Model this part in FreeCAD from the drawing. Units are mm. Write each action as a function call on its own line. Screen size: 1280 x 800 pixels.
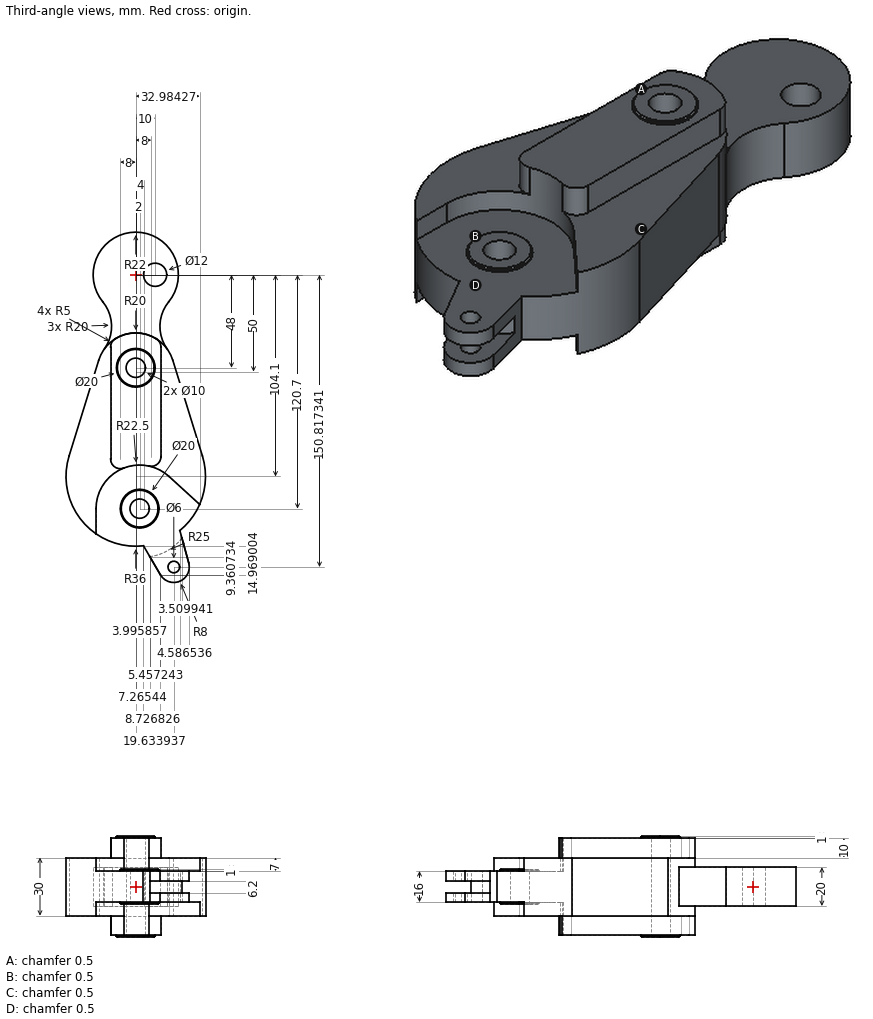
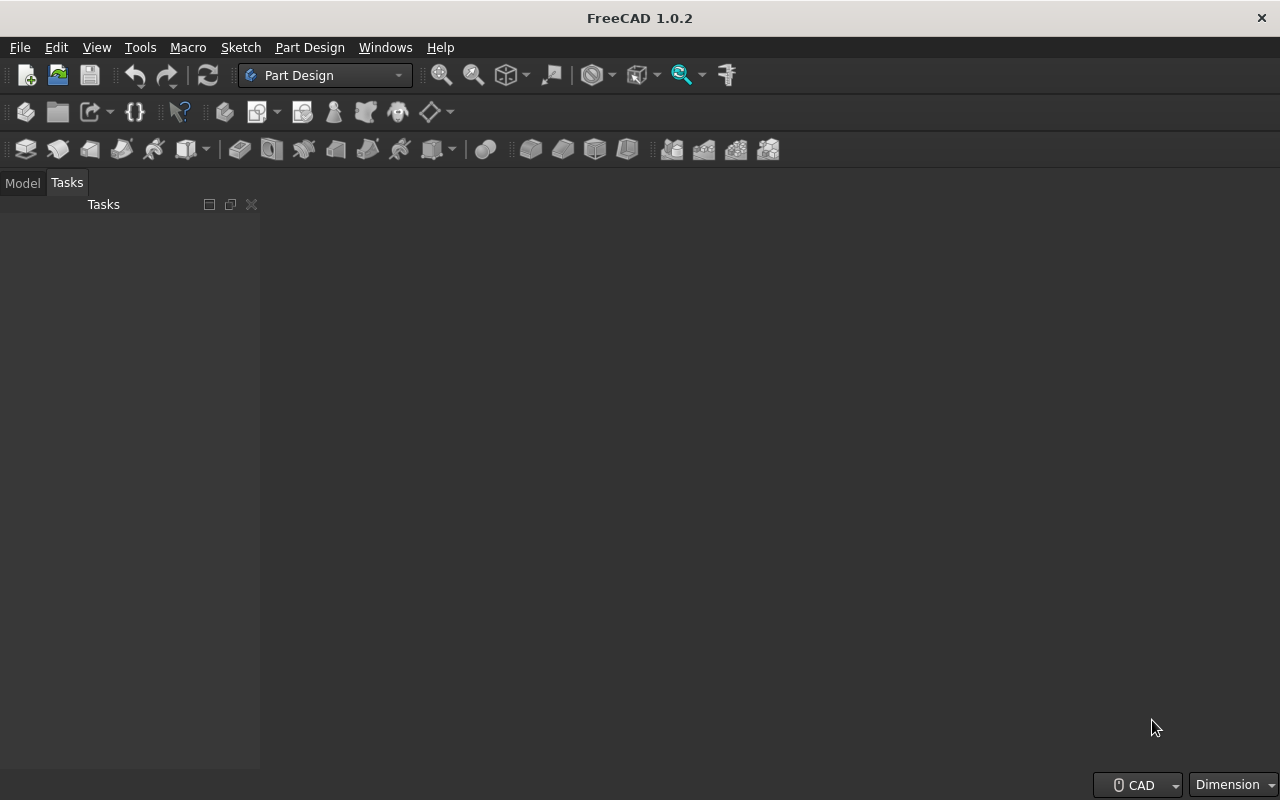
click(26, 76)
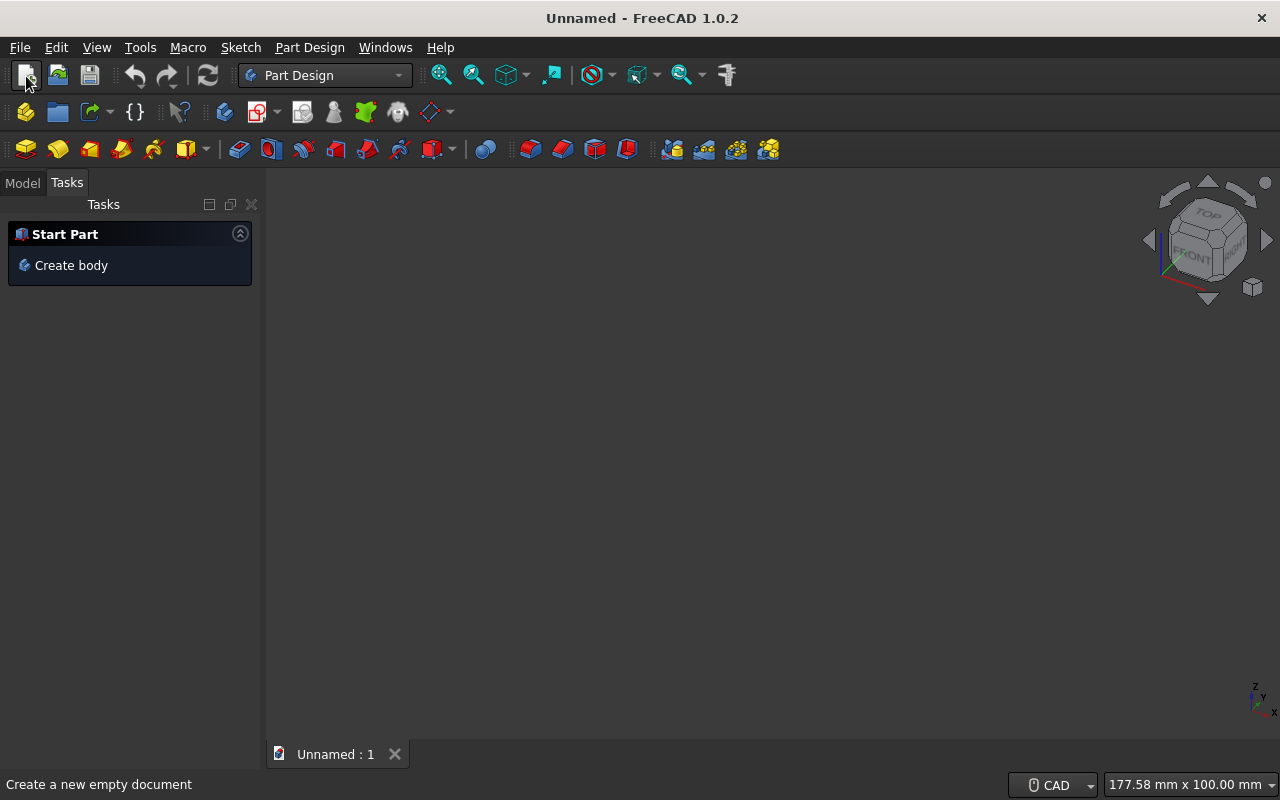
click(258, 112)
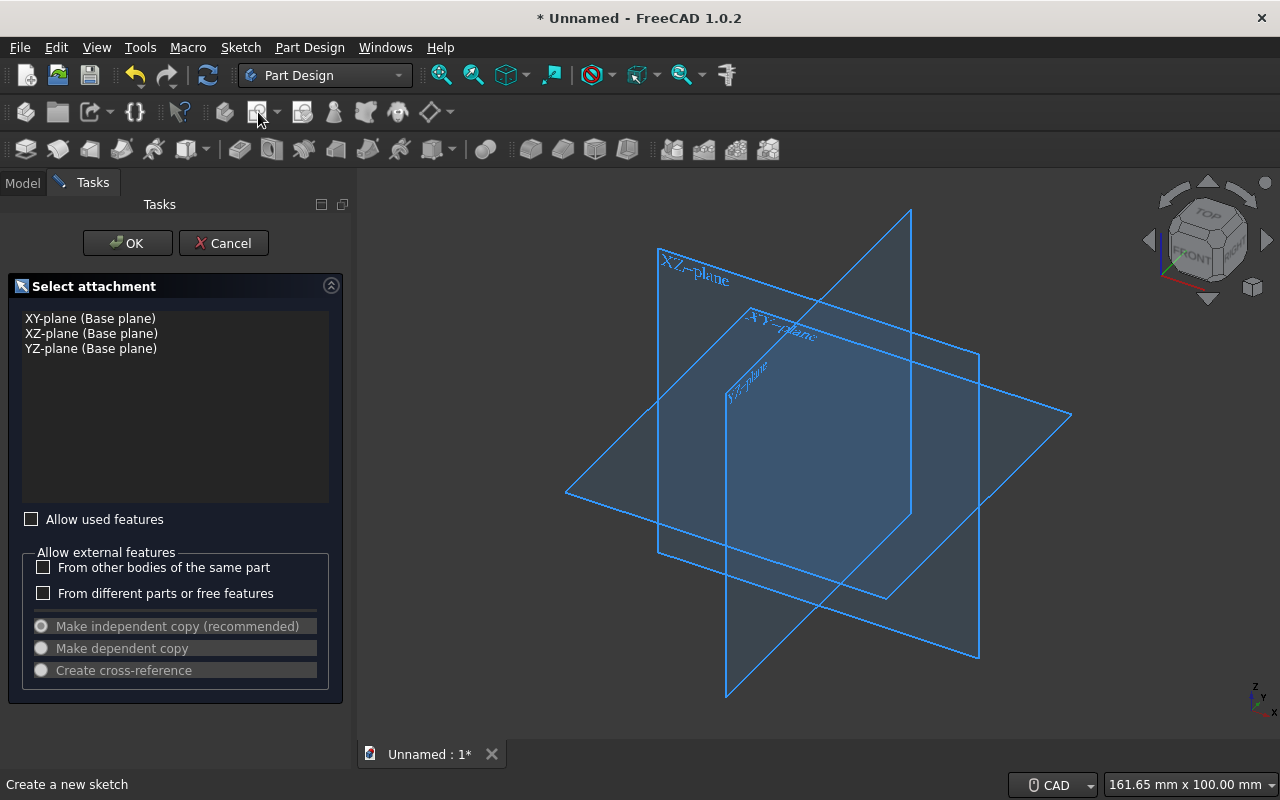
click(82, 318)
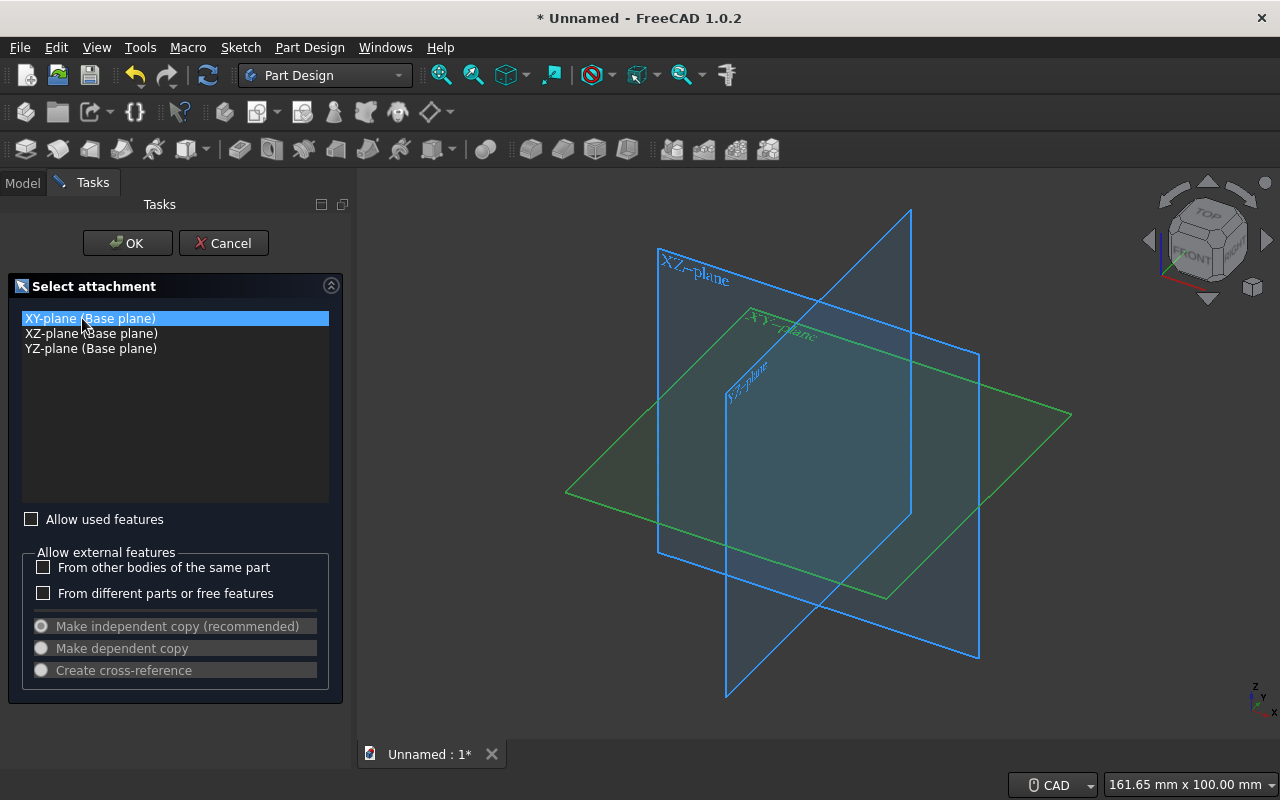
click(128, 243)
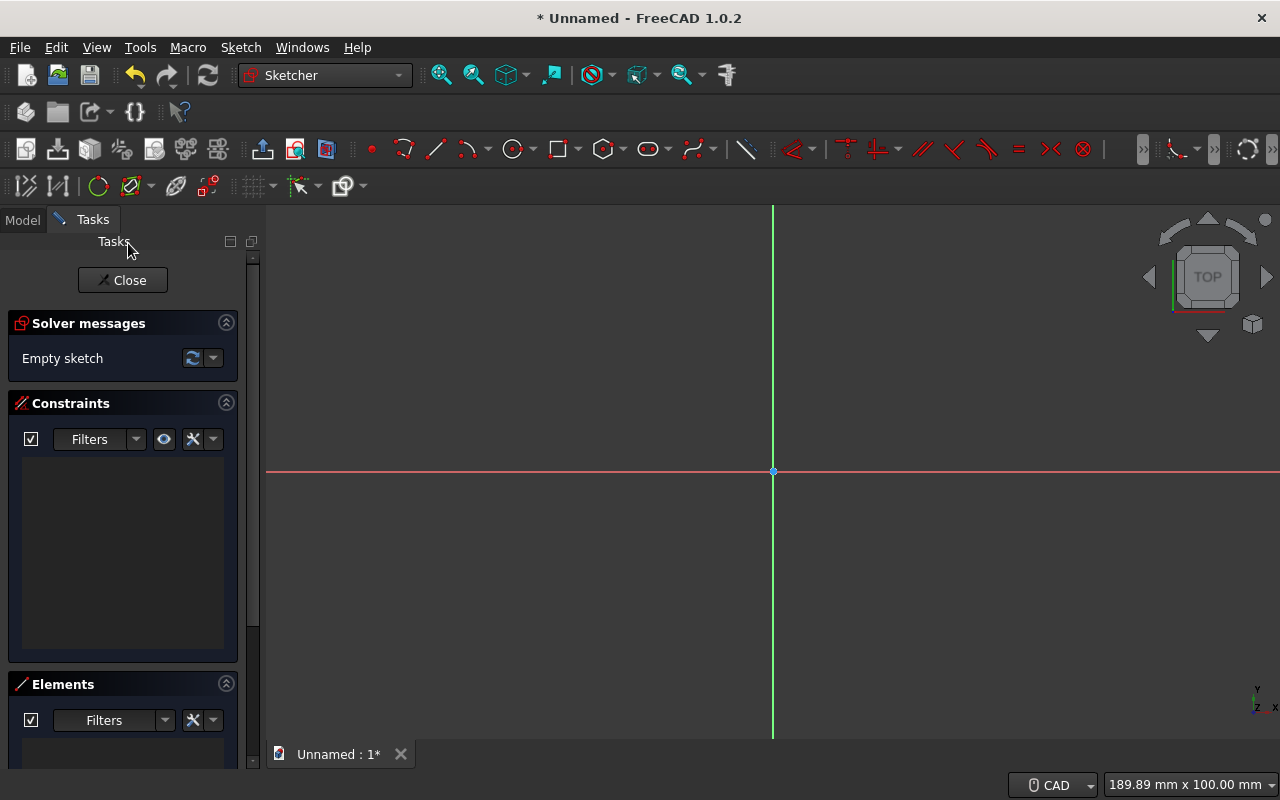
click(490, 150)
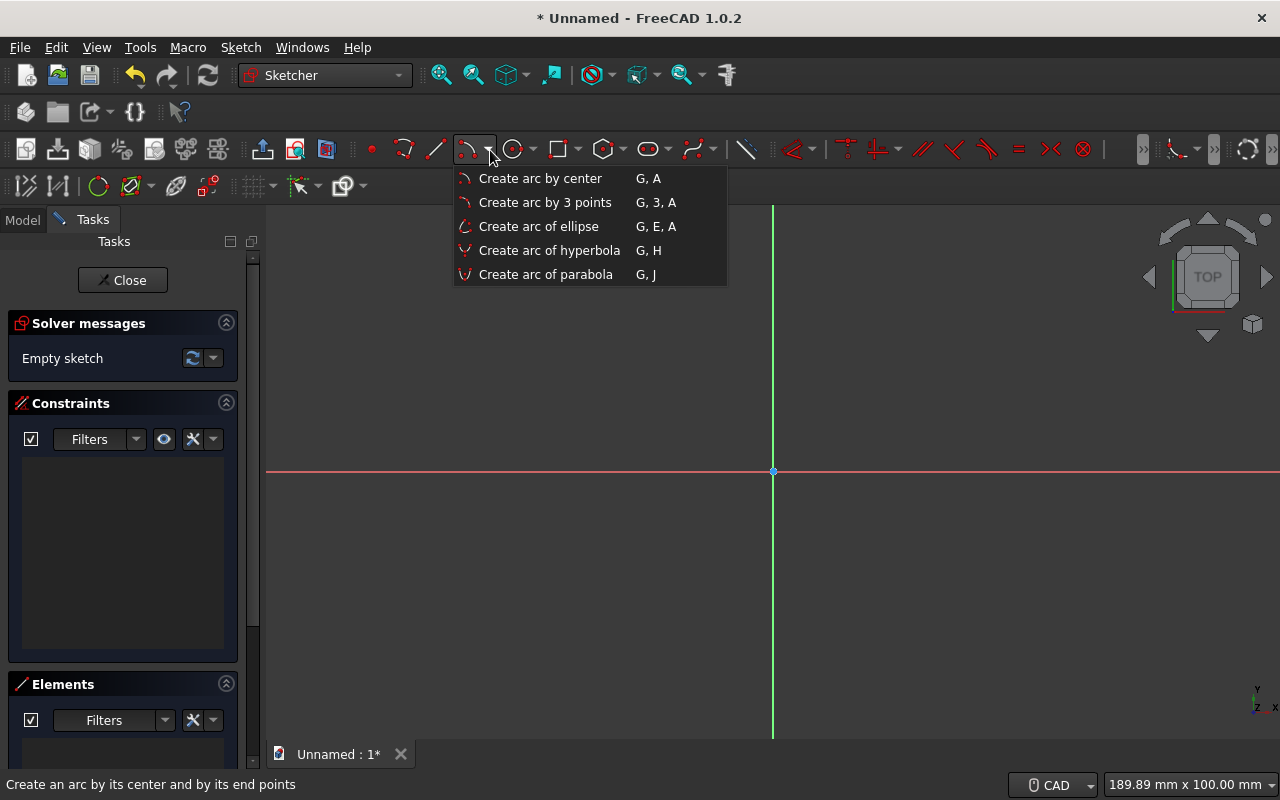
click(590, 202)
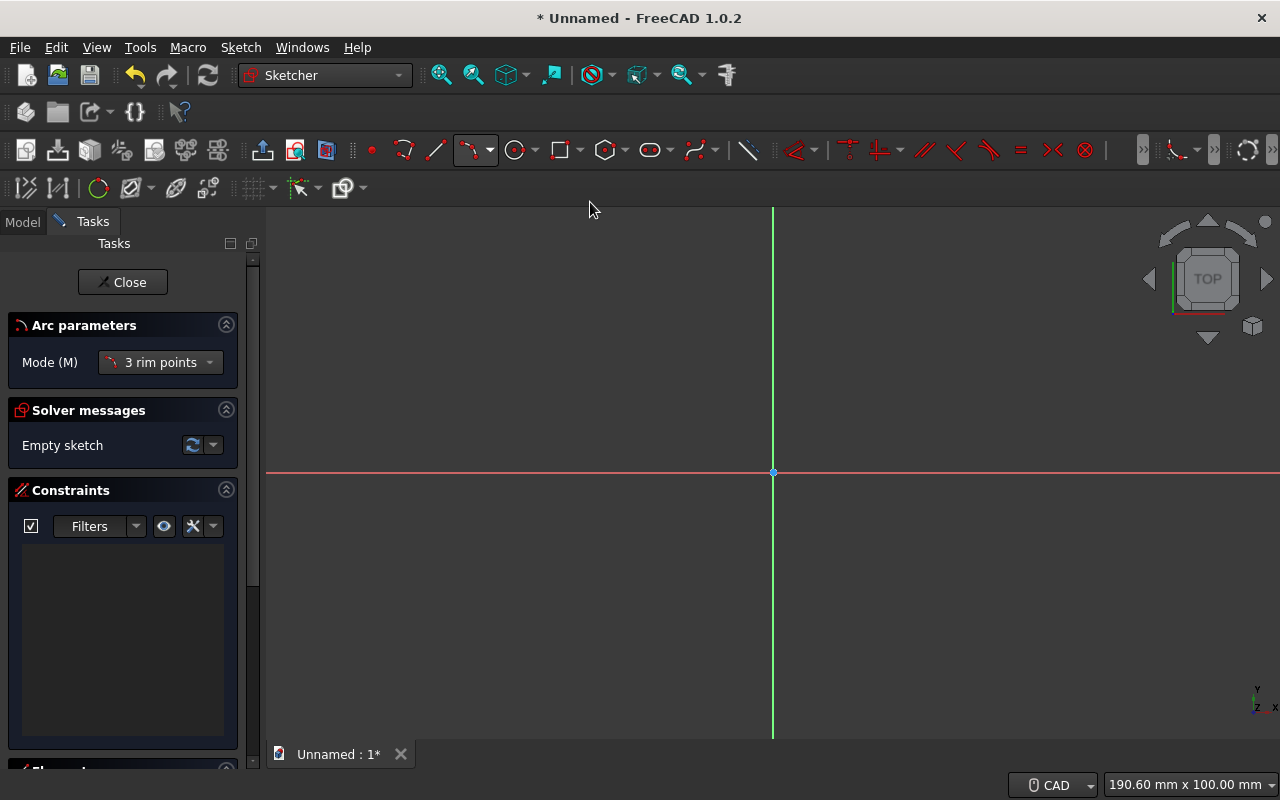
click(683, 547)
click(687, 677)
click(707, 611)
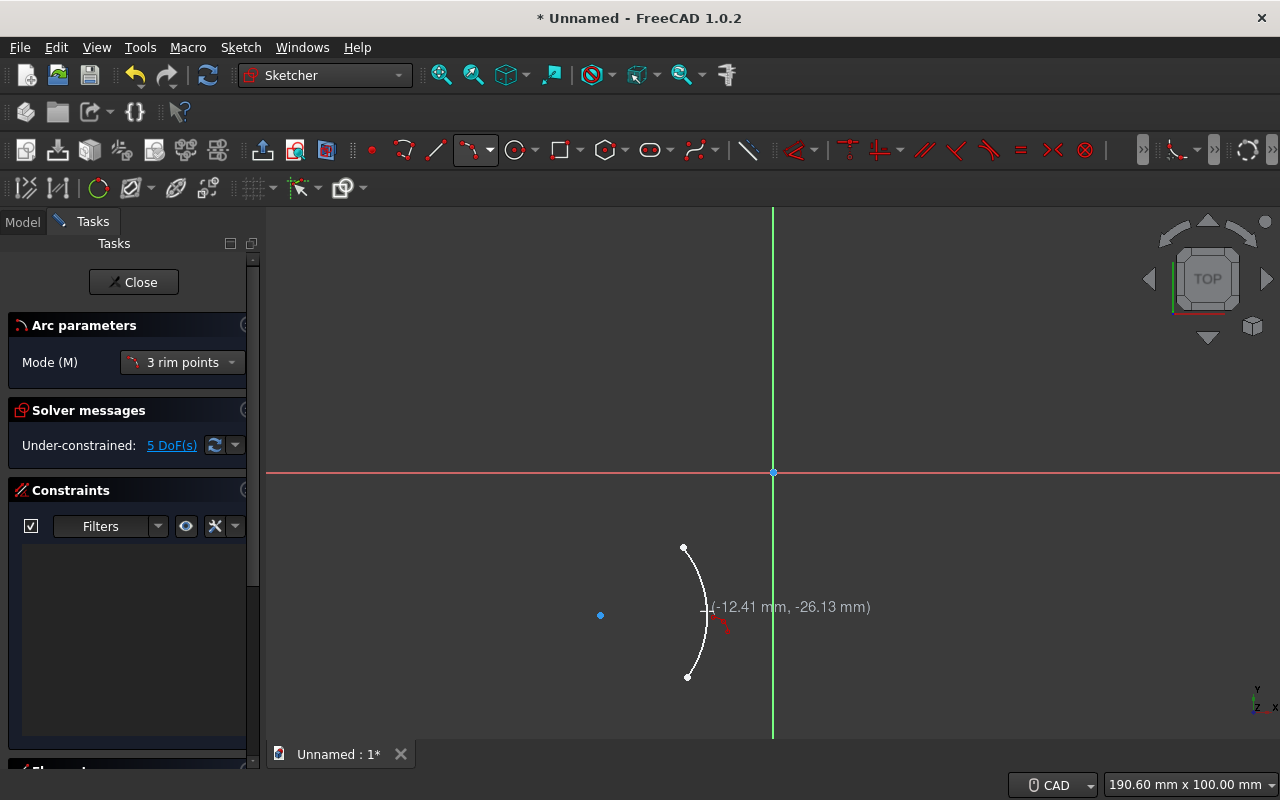
click(687, 678)
click(859, 677)
click(793, 635)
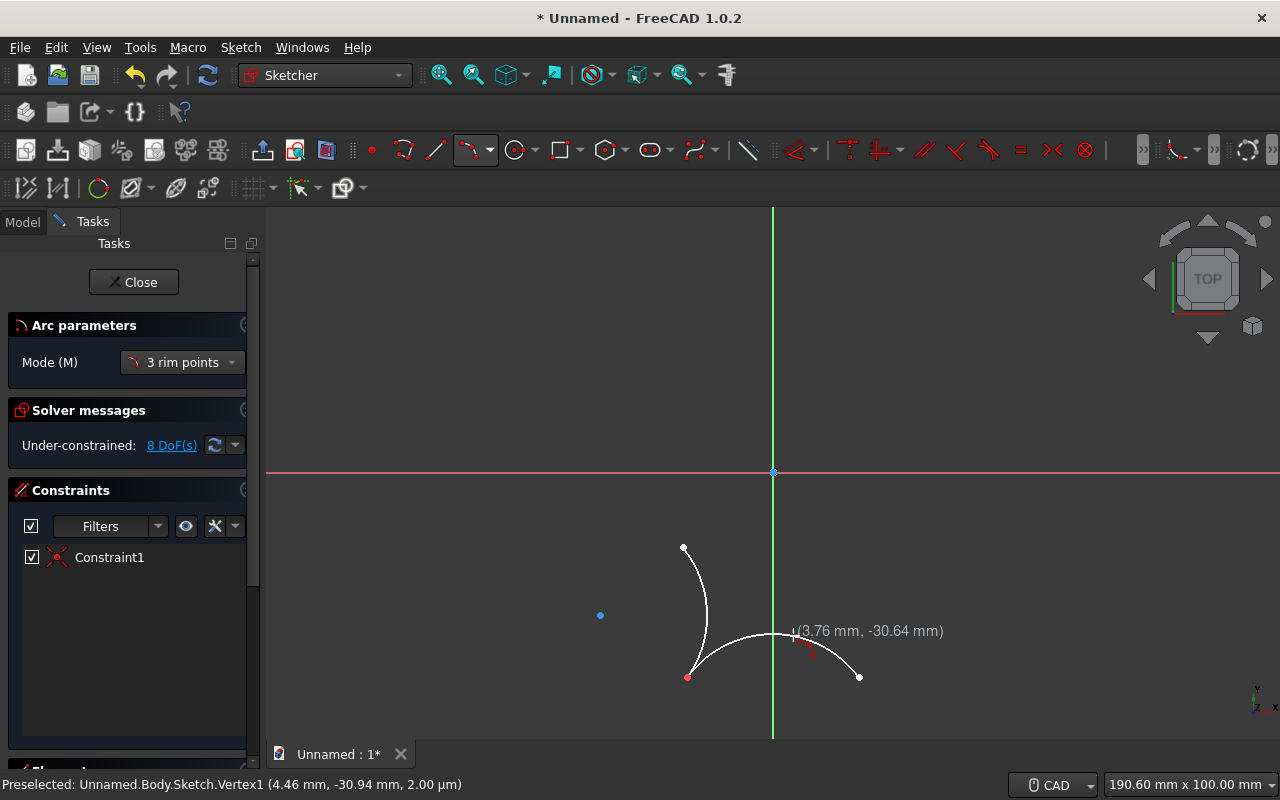
click(859, 678)
click(863, 547)
click(839, 611)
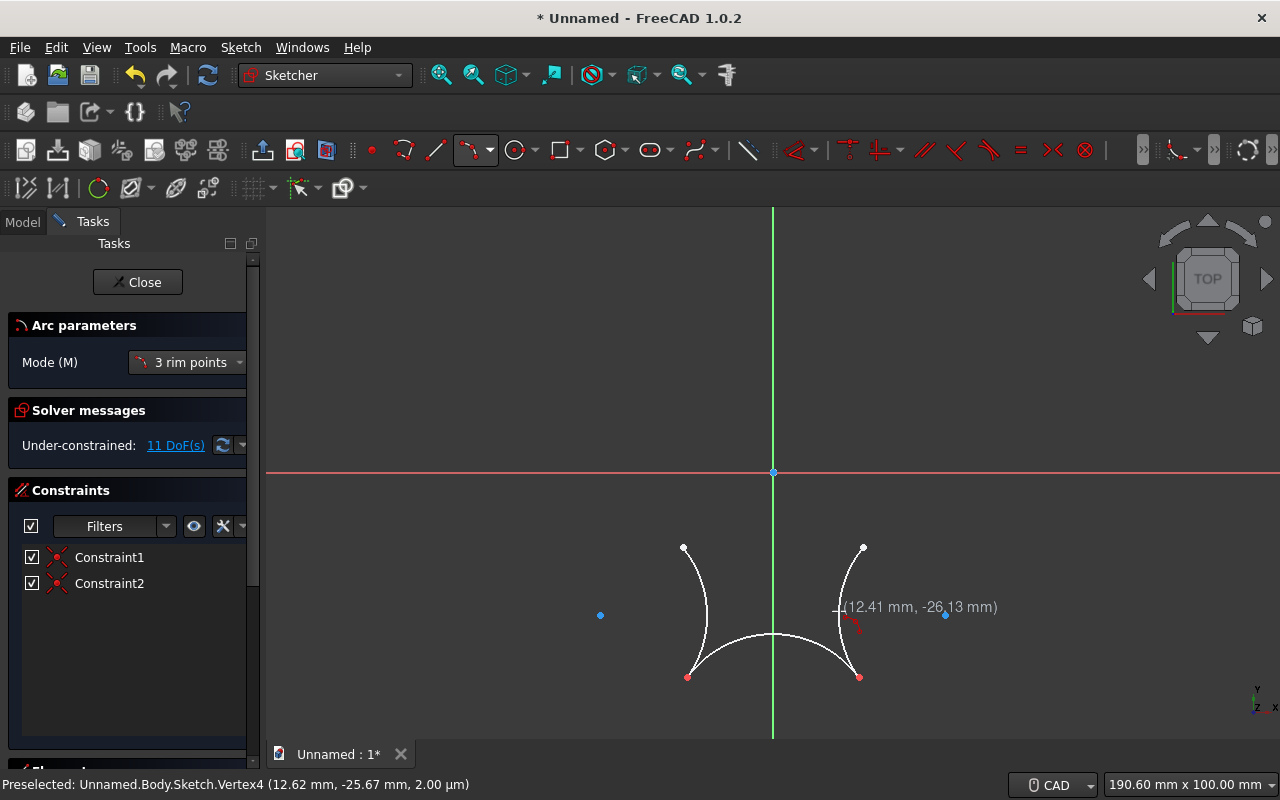
click(863, 548)
click(683, 548)
click(824, 368)